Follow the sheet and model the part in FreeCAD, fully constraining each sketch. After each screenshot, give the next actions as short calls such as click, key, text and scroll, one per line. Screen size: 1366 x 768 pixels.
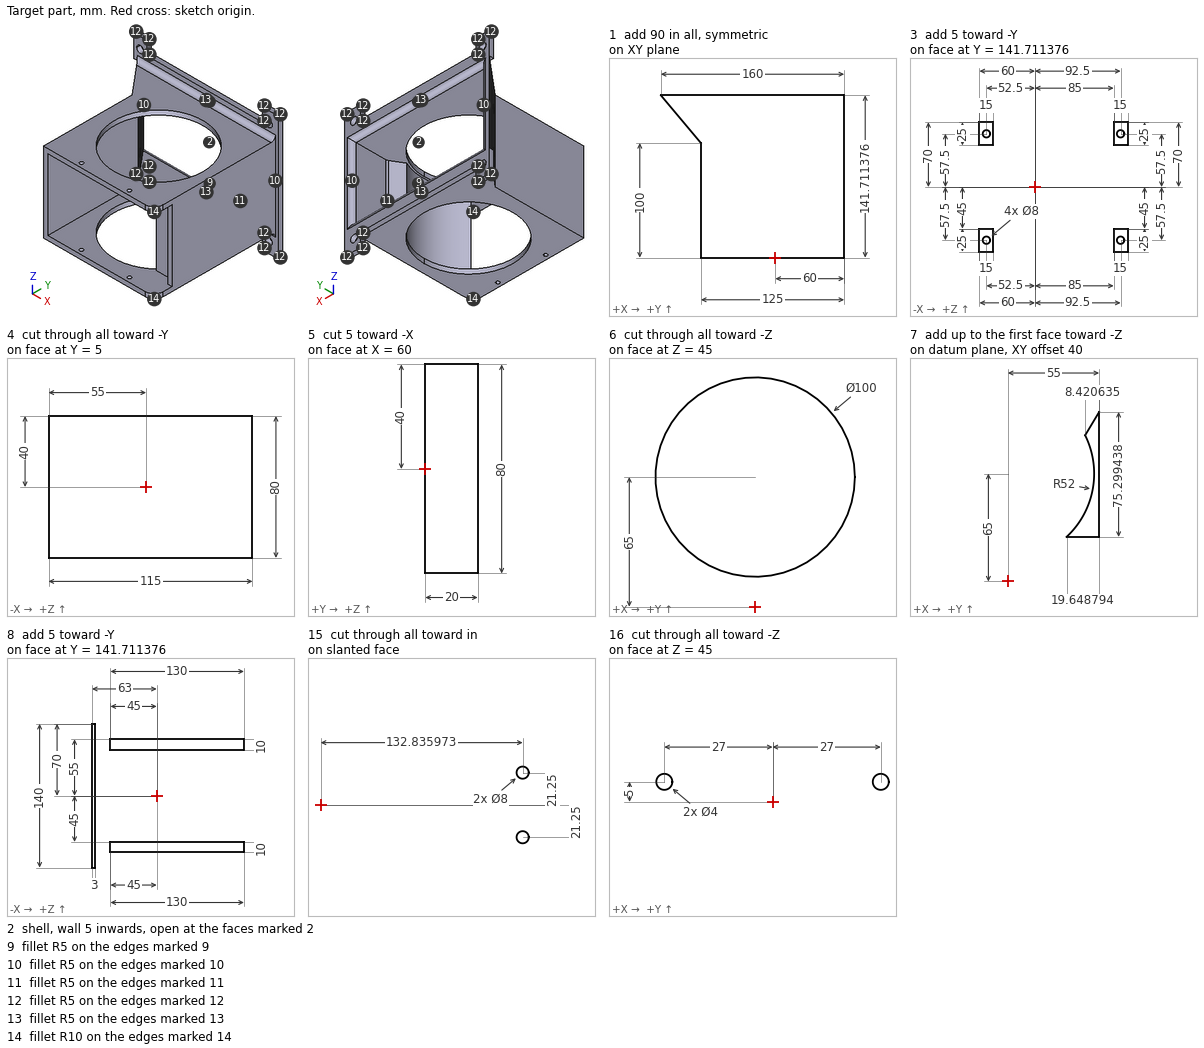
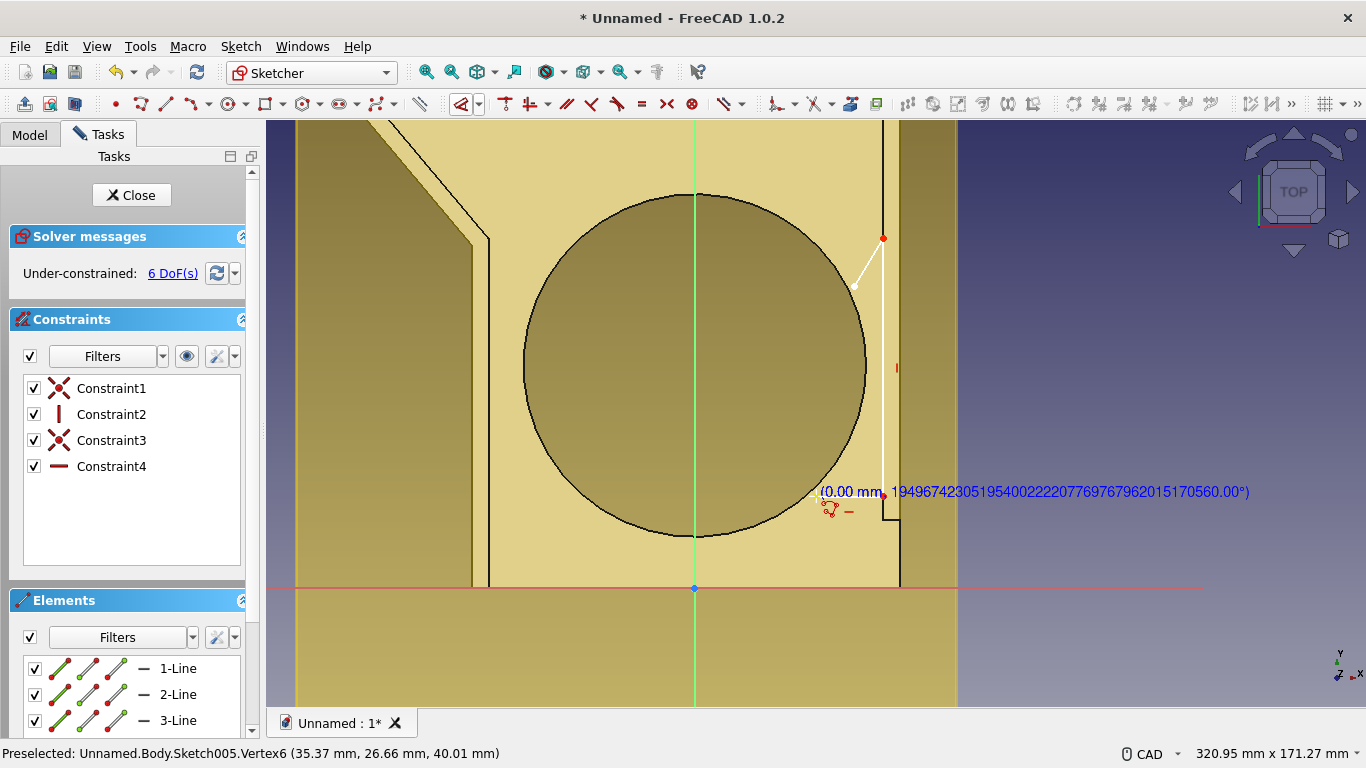
key(g)
key(3)
key(a)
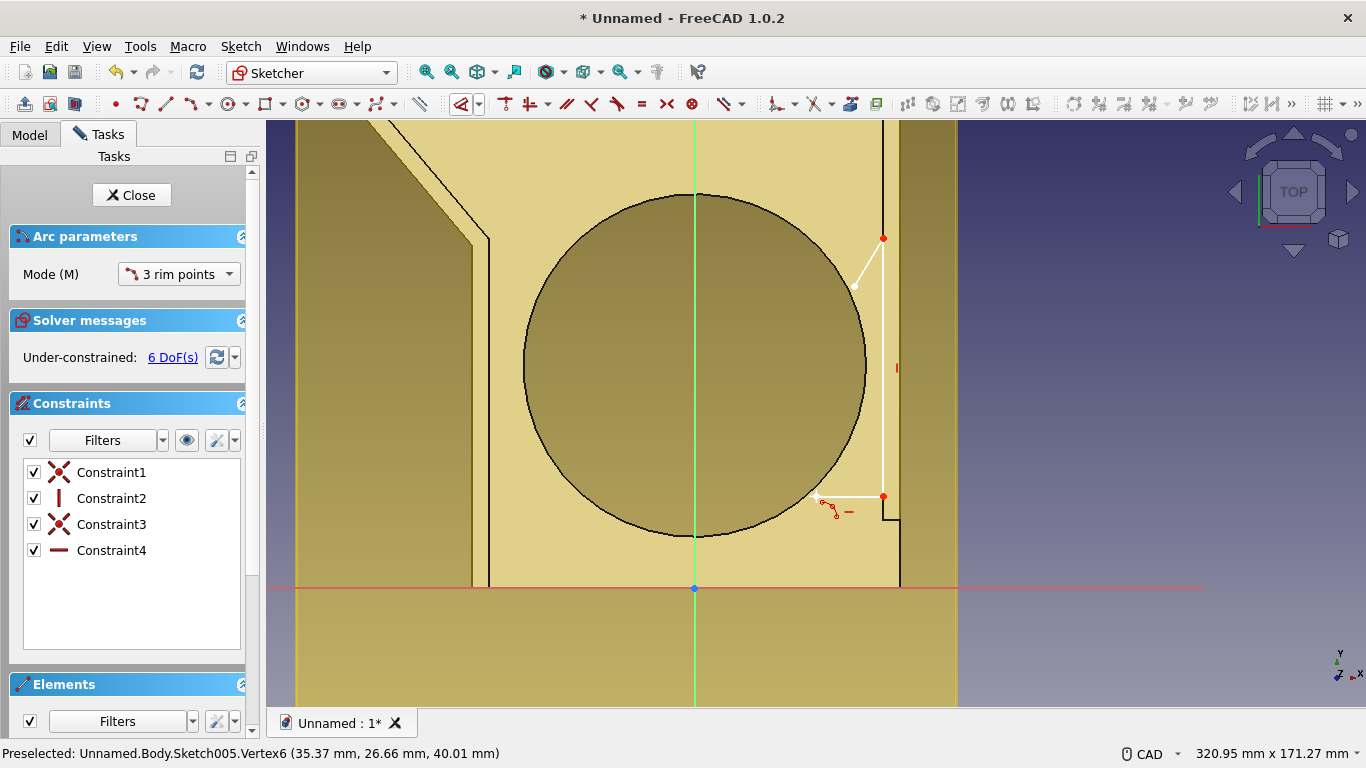
click(816, 497)
click(854, 287)
click(865, 420)
key(Escape)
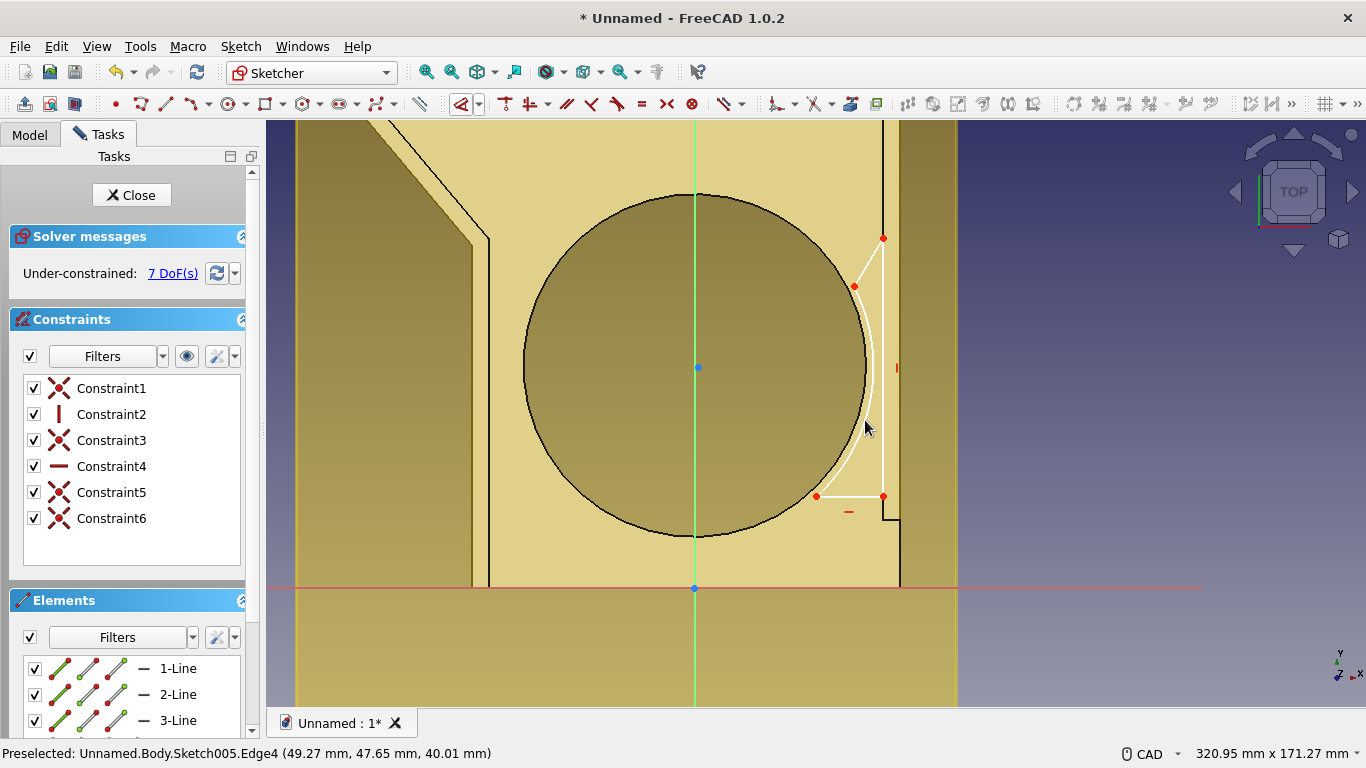
click(698, 367)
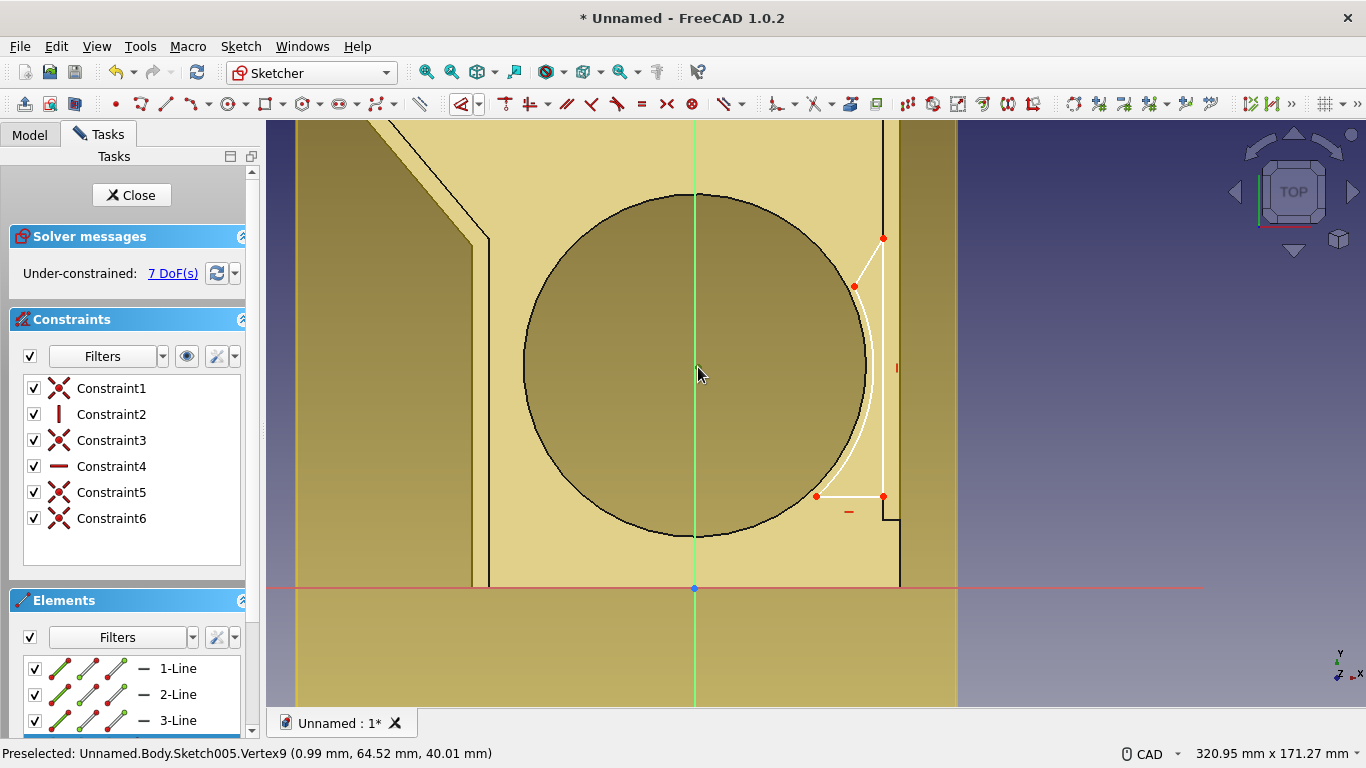
click(695, 641)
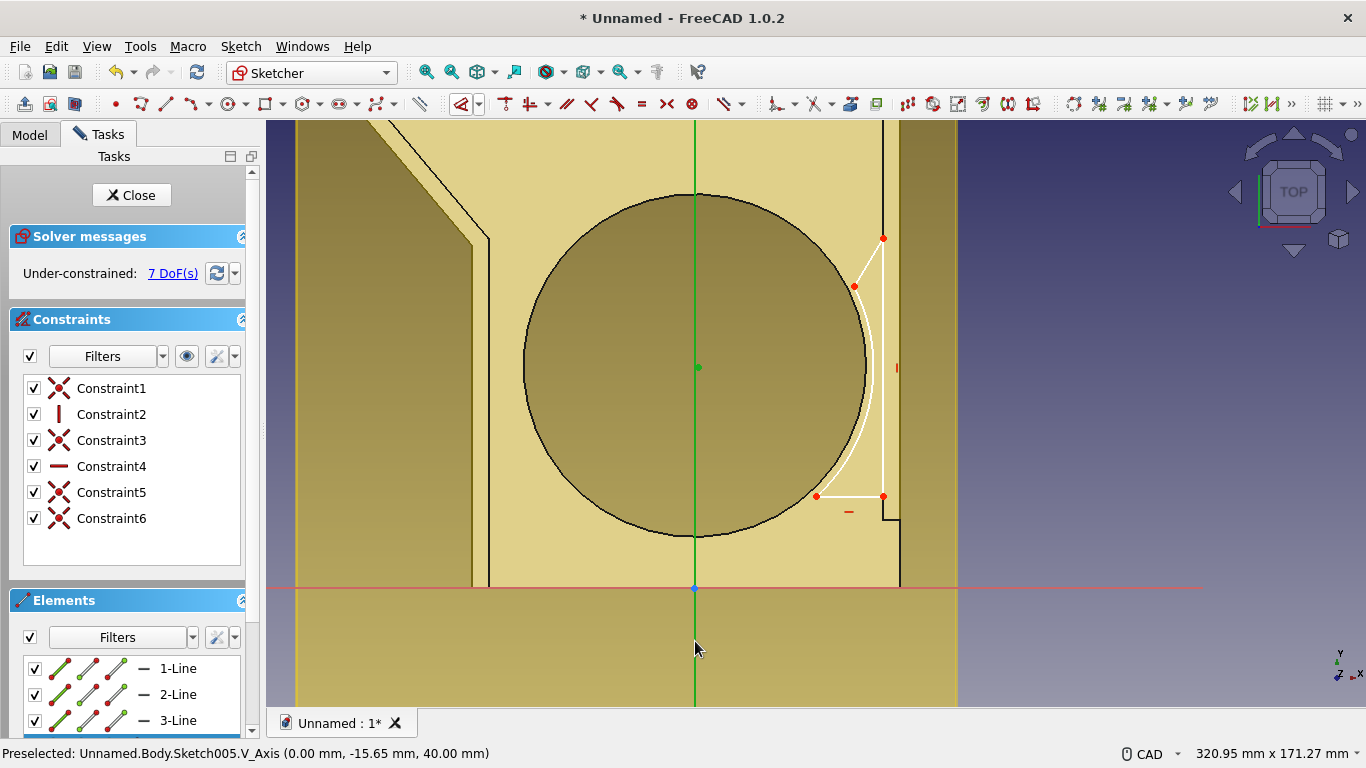
key(c)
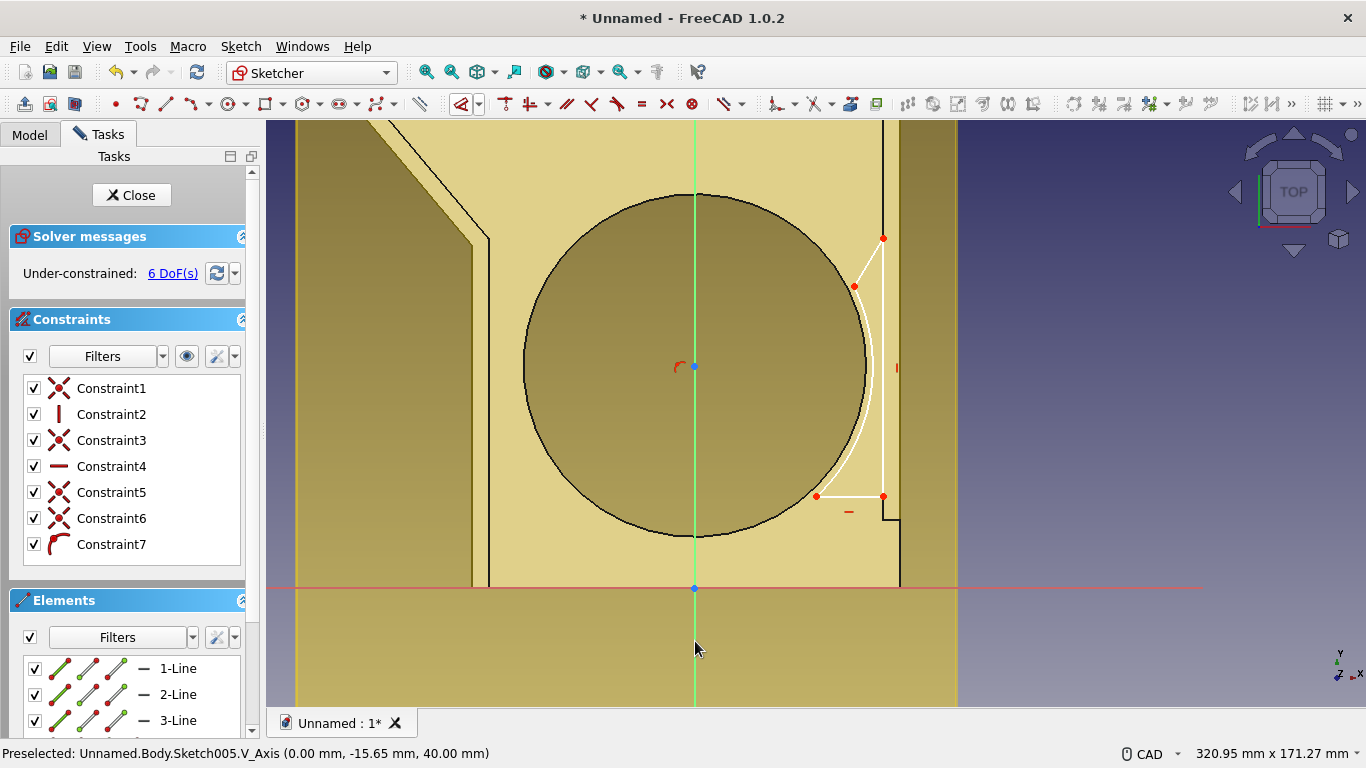
click(856, 442)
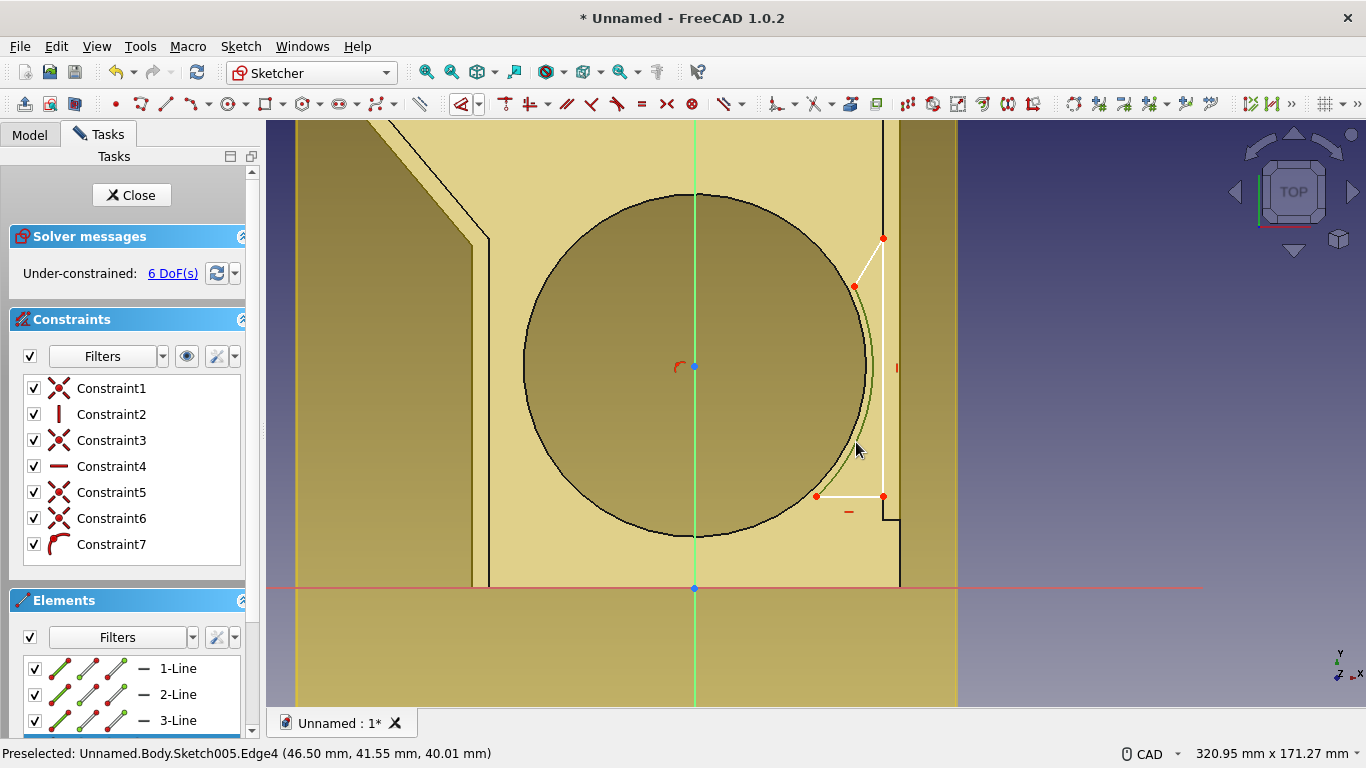
key(k)
key(r)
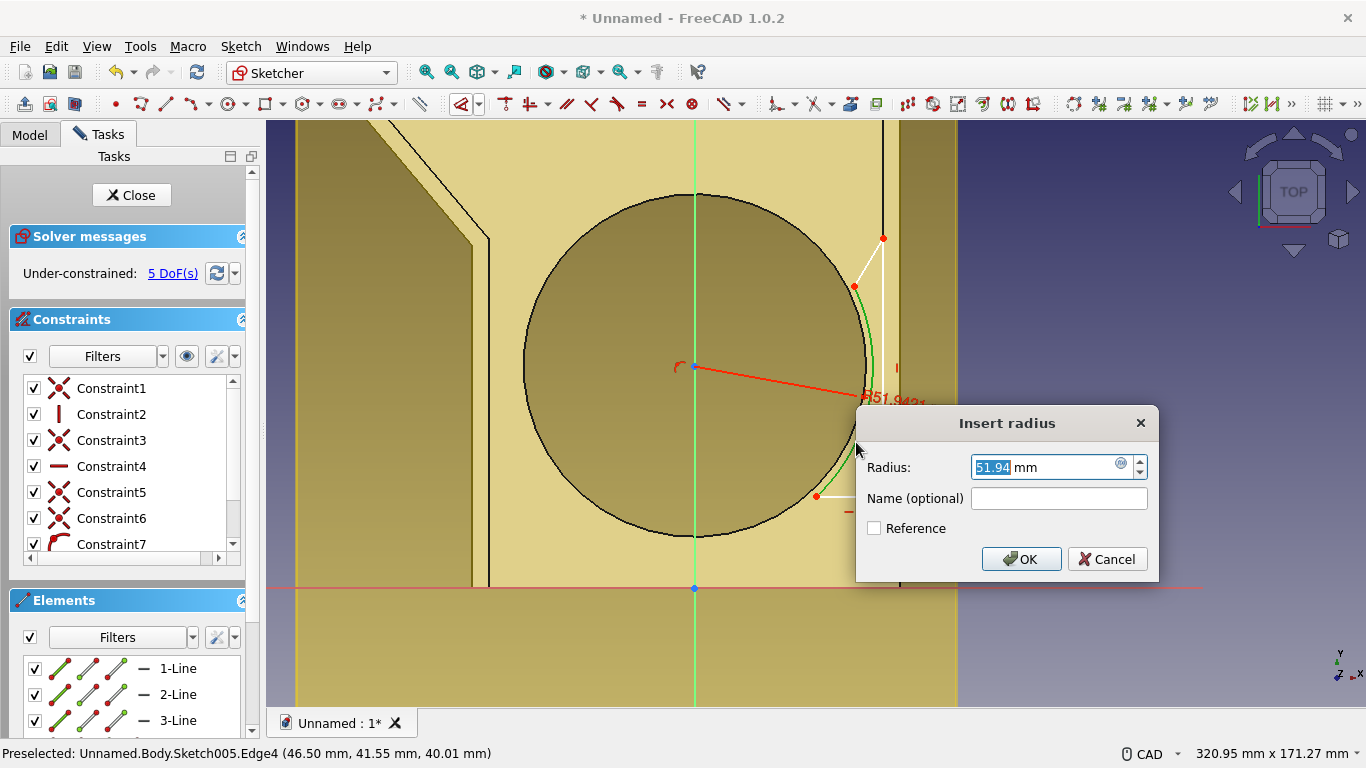
text(52)
key(Return)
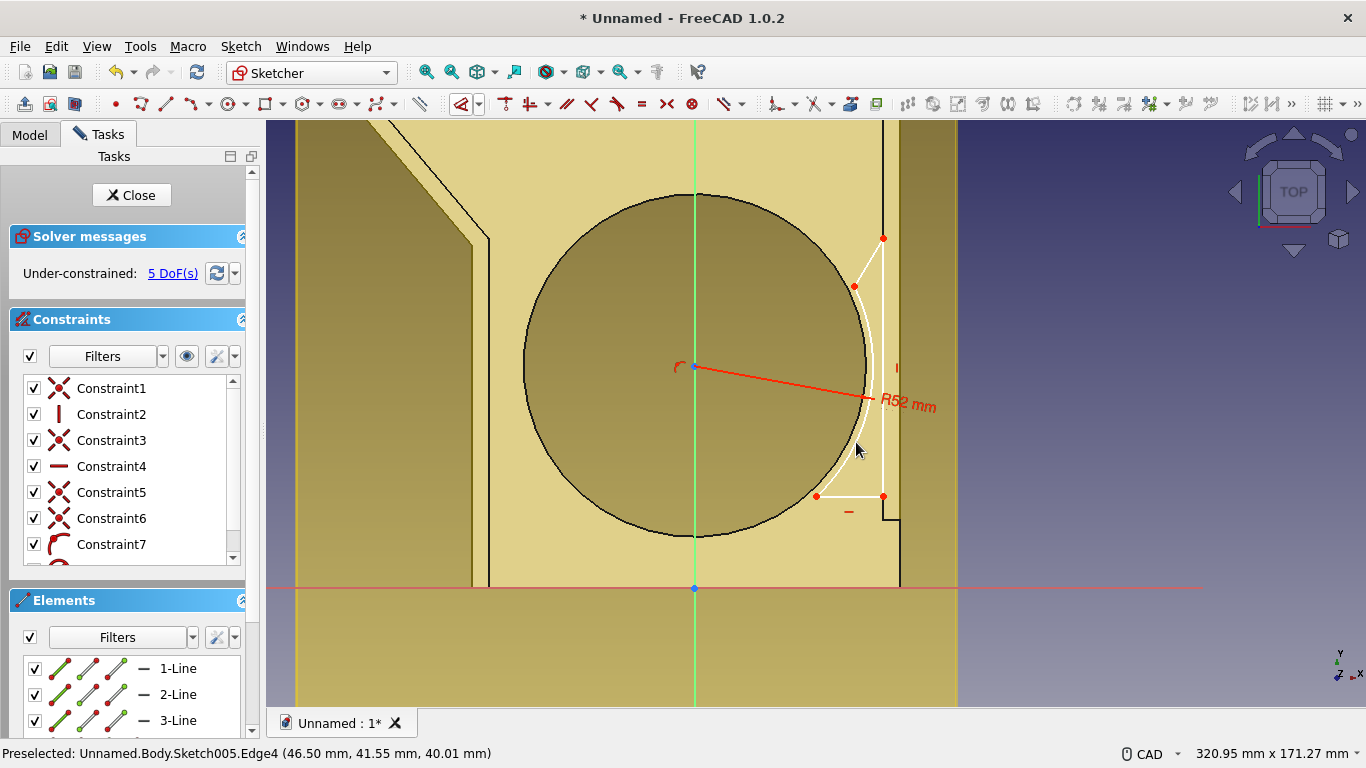
click(883, 239)